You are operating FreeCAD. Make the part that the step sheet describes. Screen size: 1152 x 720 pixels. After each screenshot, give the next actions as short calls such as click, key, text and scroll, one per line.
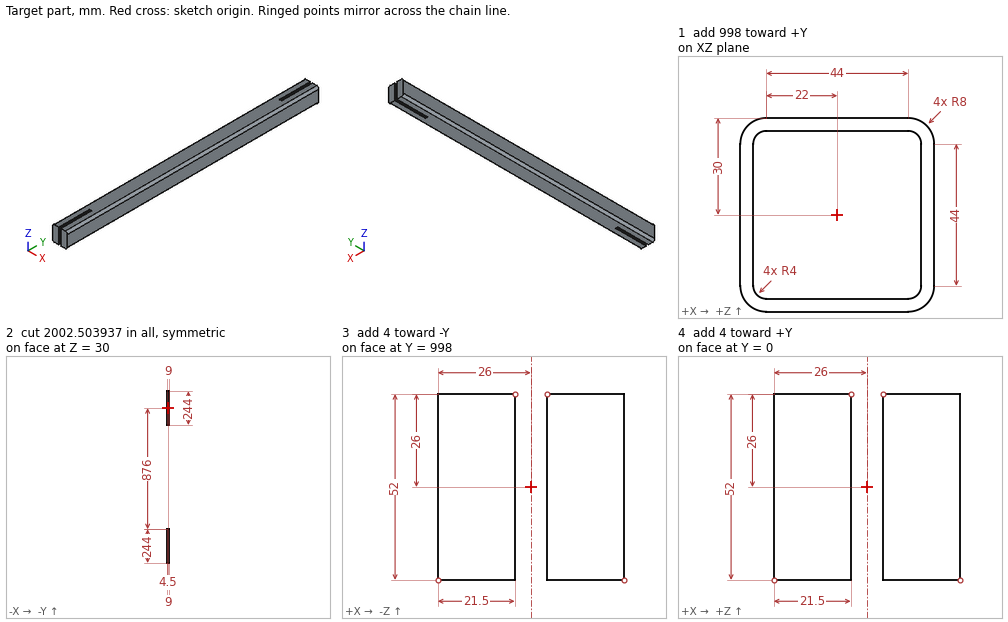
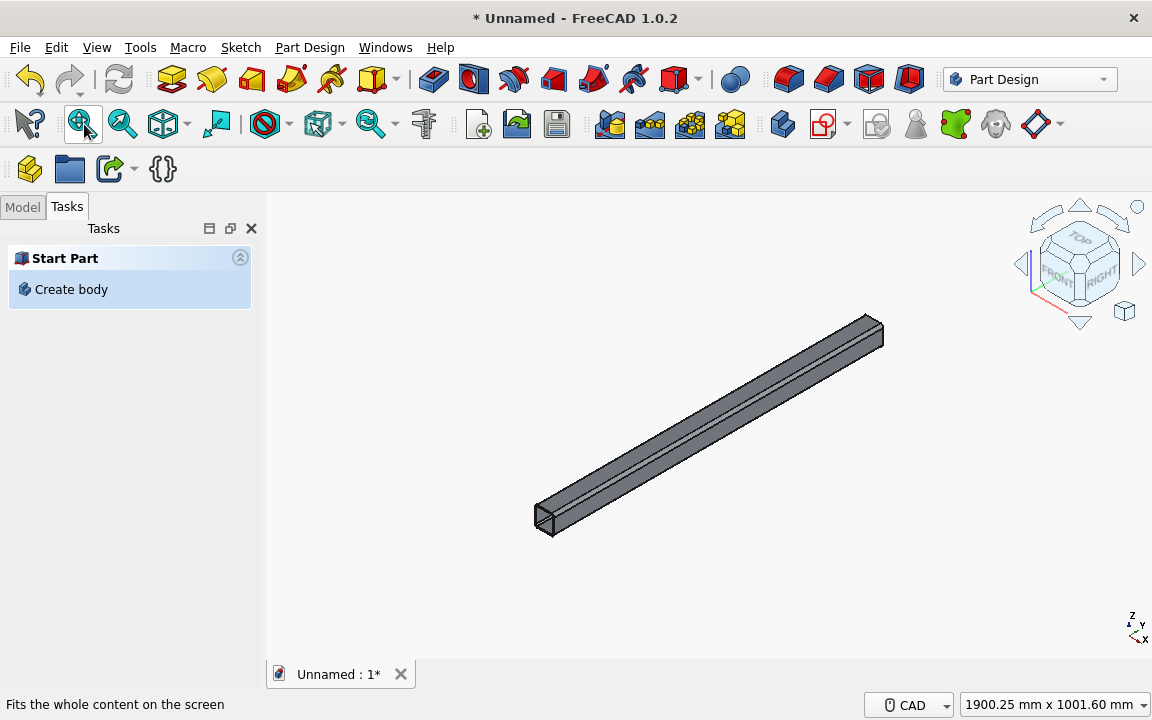
key(2)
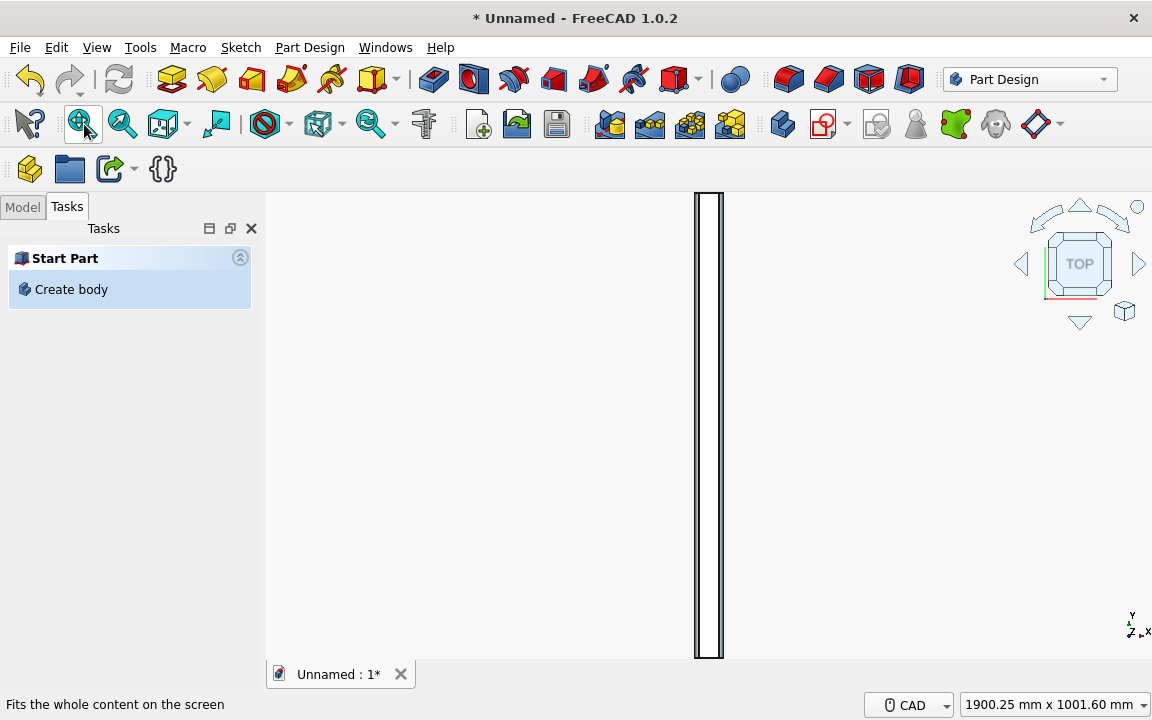
click(709, 225)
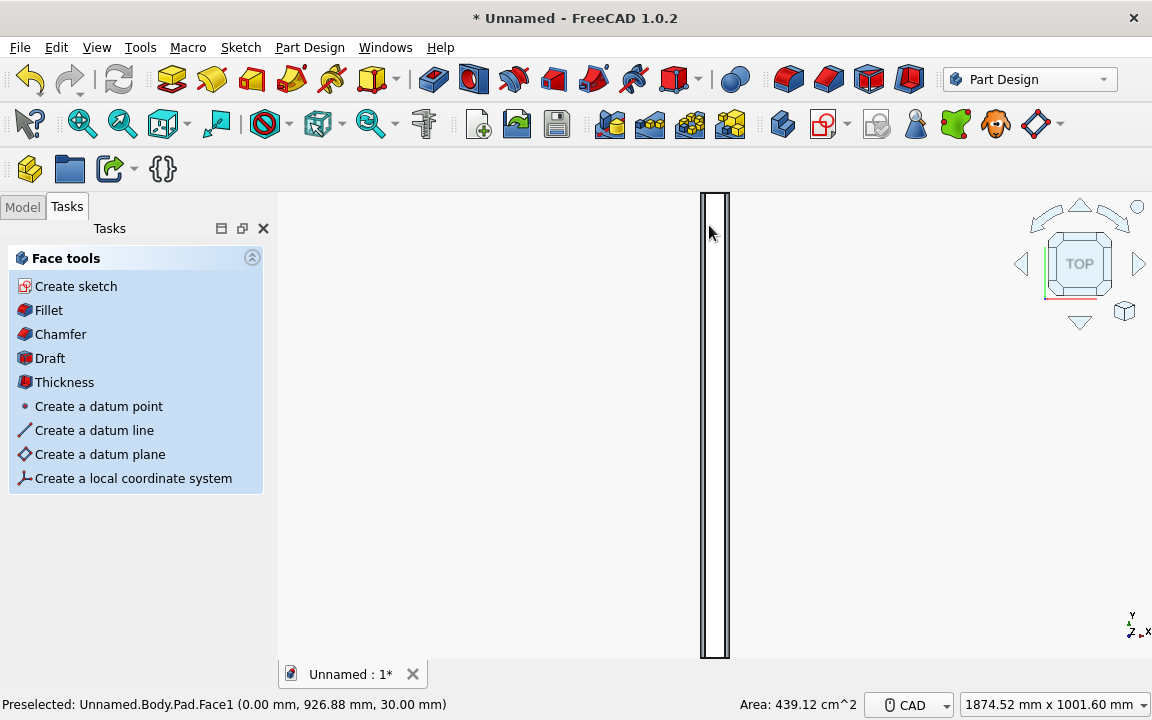
click(824, 124)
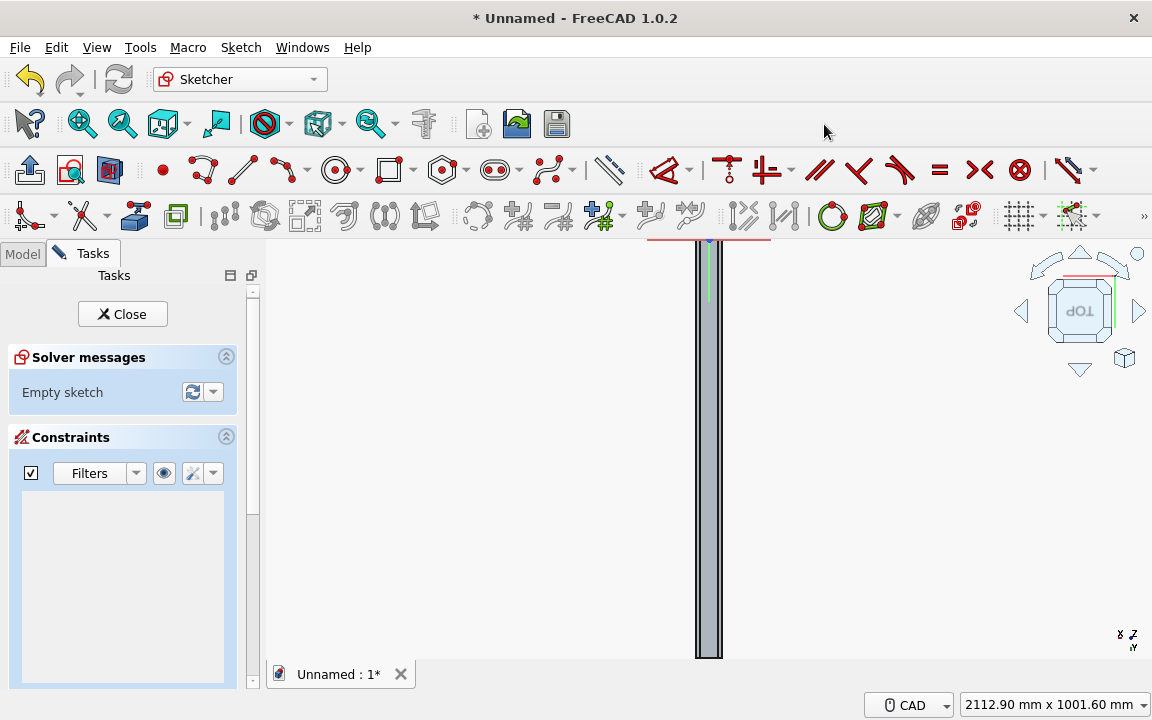
scroll(585, 449, down, 4)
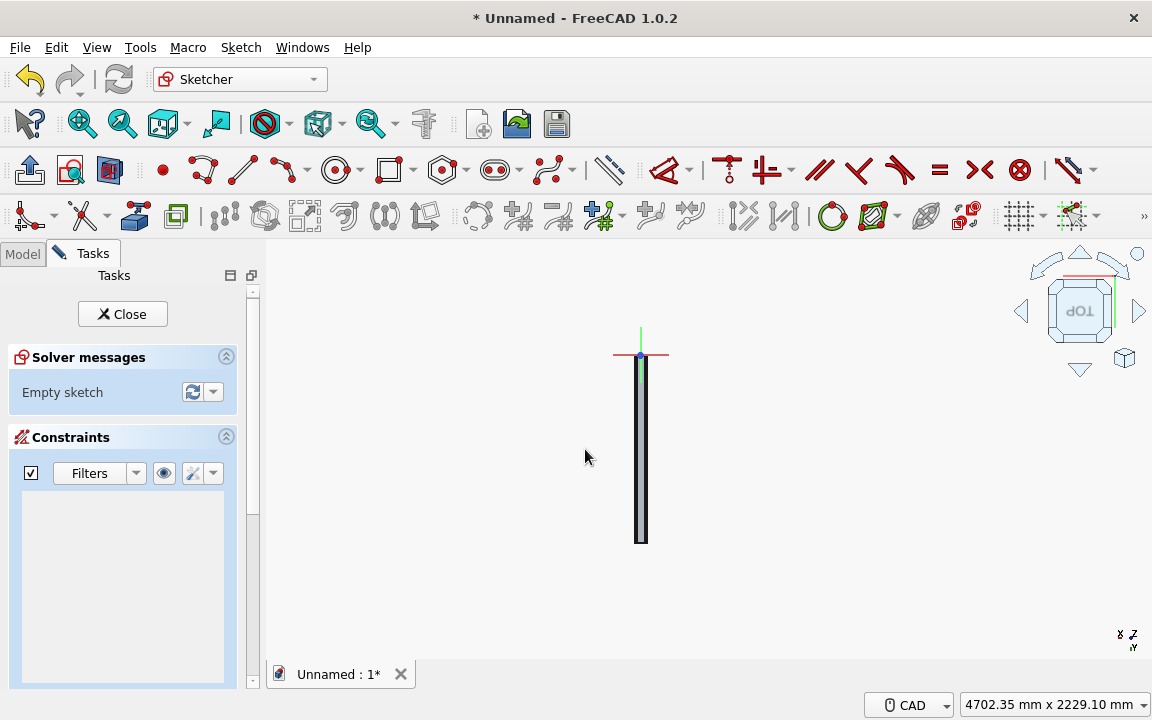
click(390, 170)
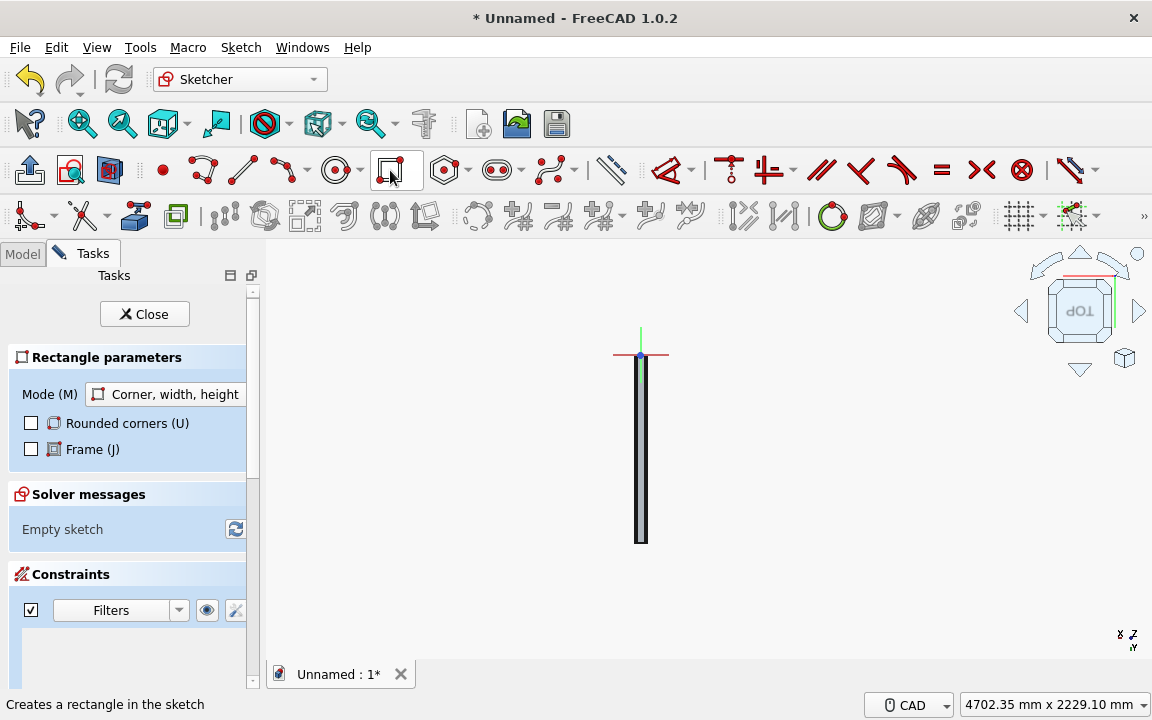
scroll(640, 520, up, 15)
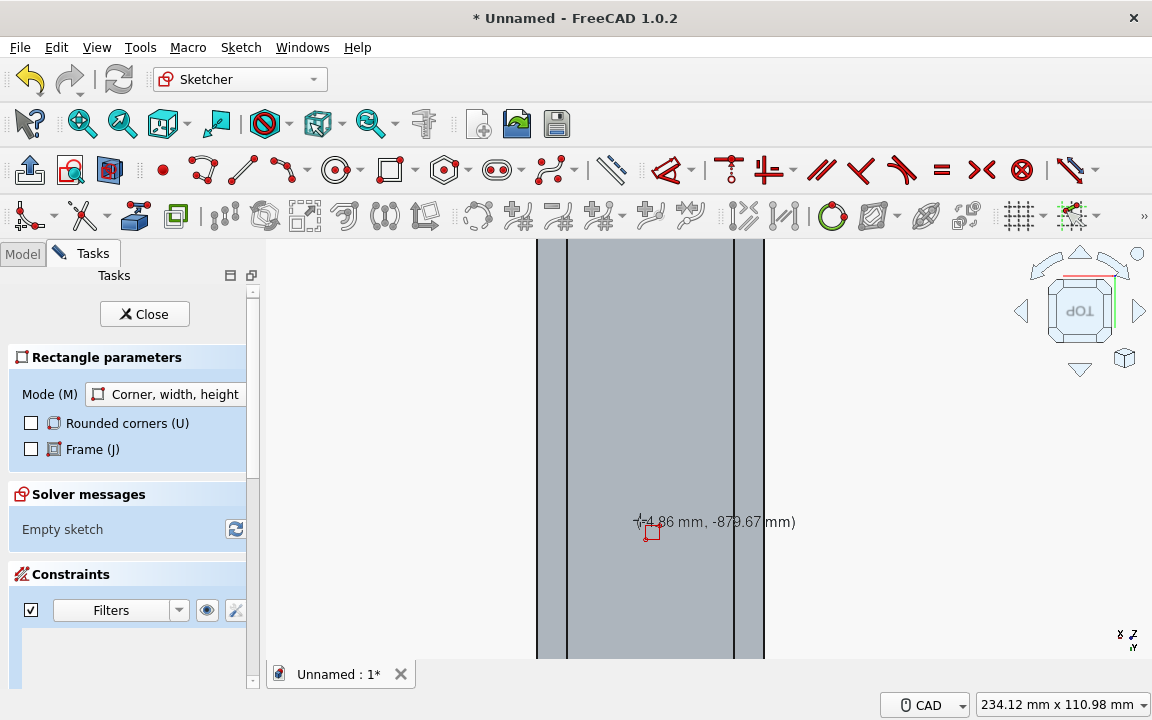
click(633, 513)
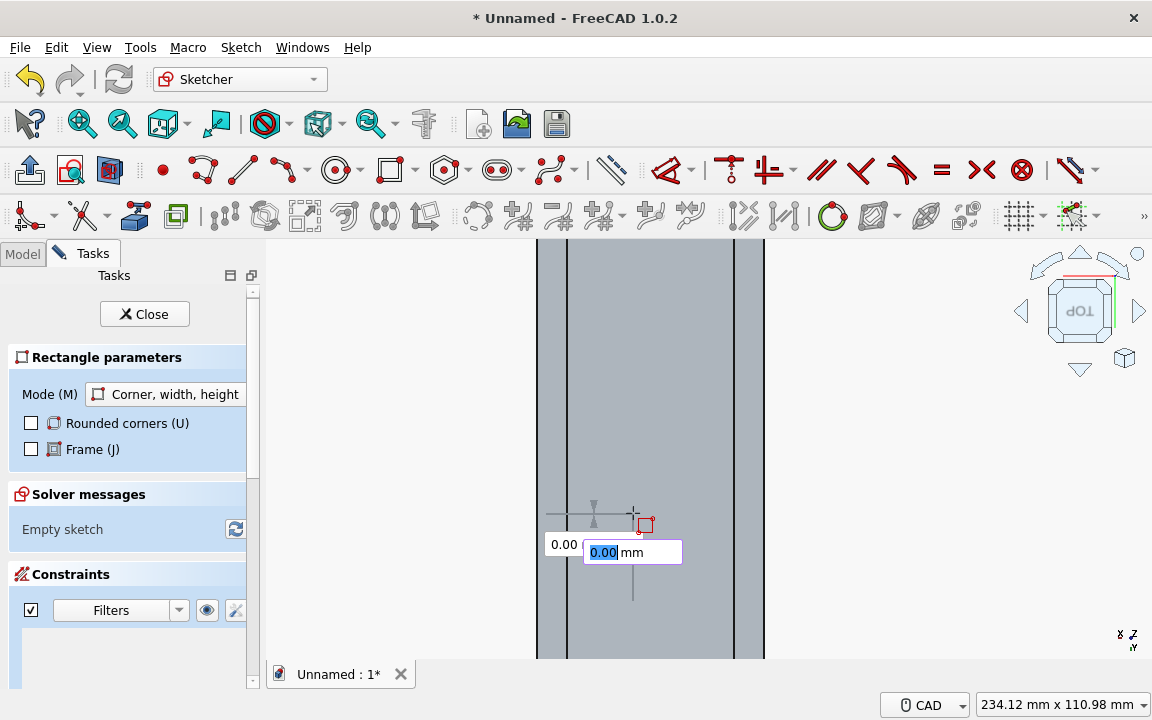
scroll(640, 520, down, 15)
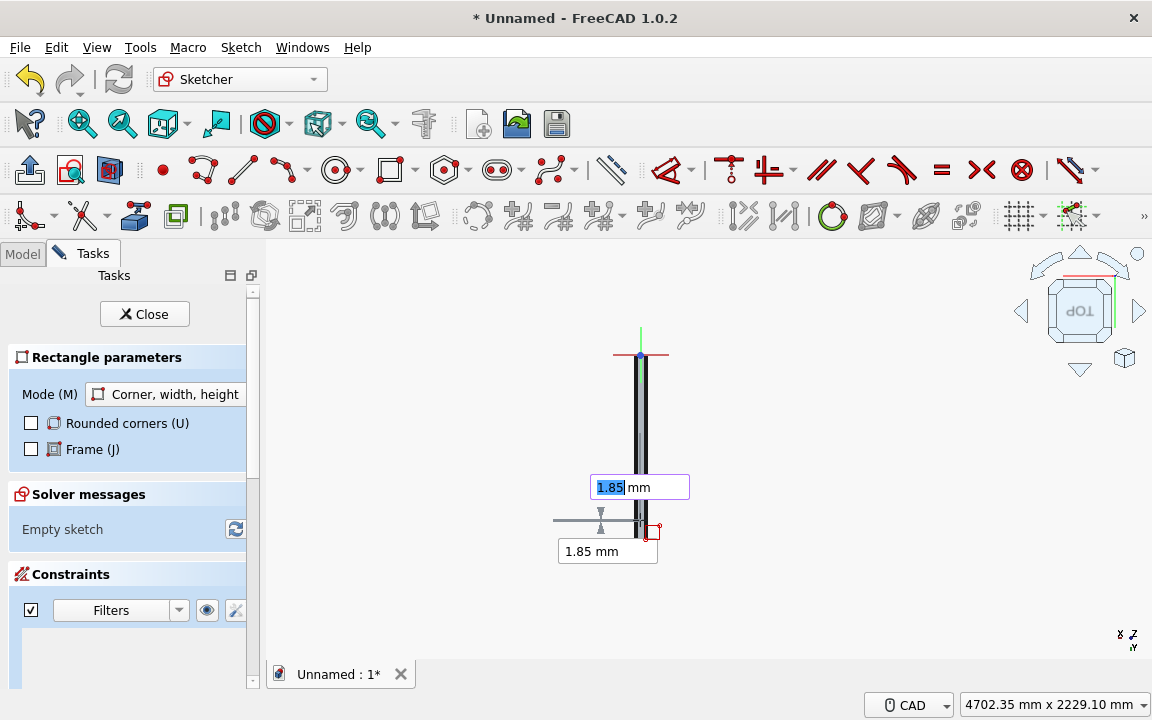
scroll(642, 566, up, 15)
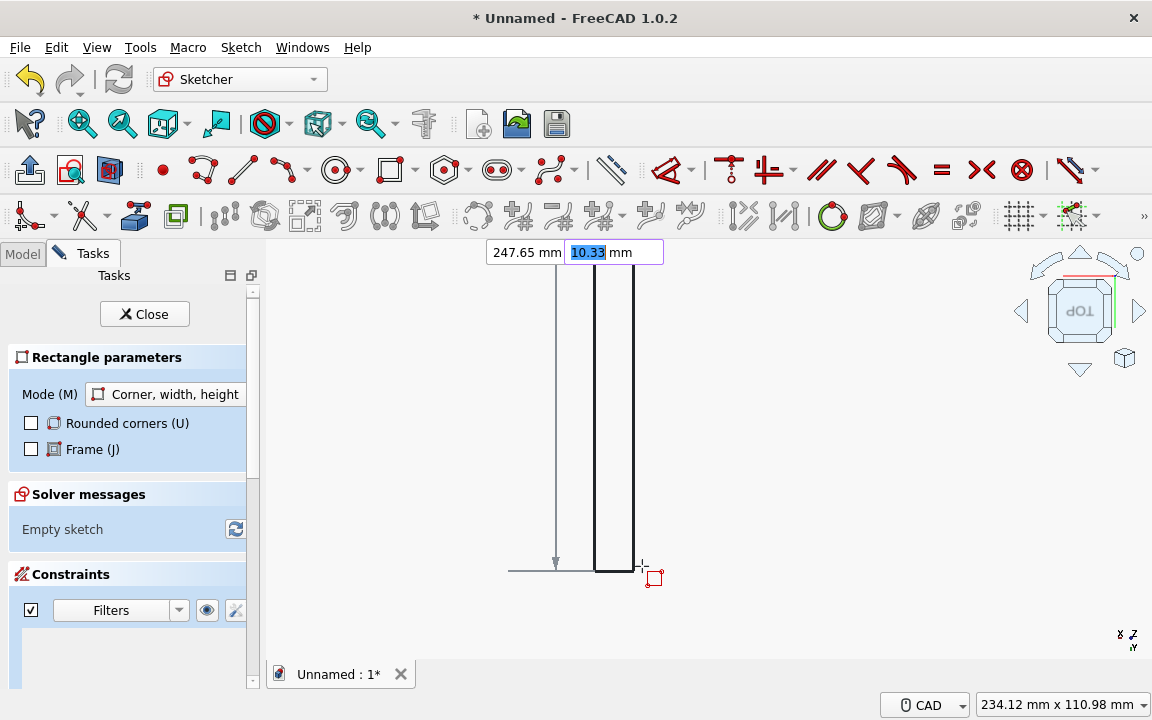
click(629, 557)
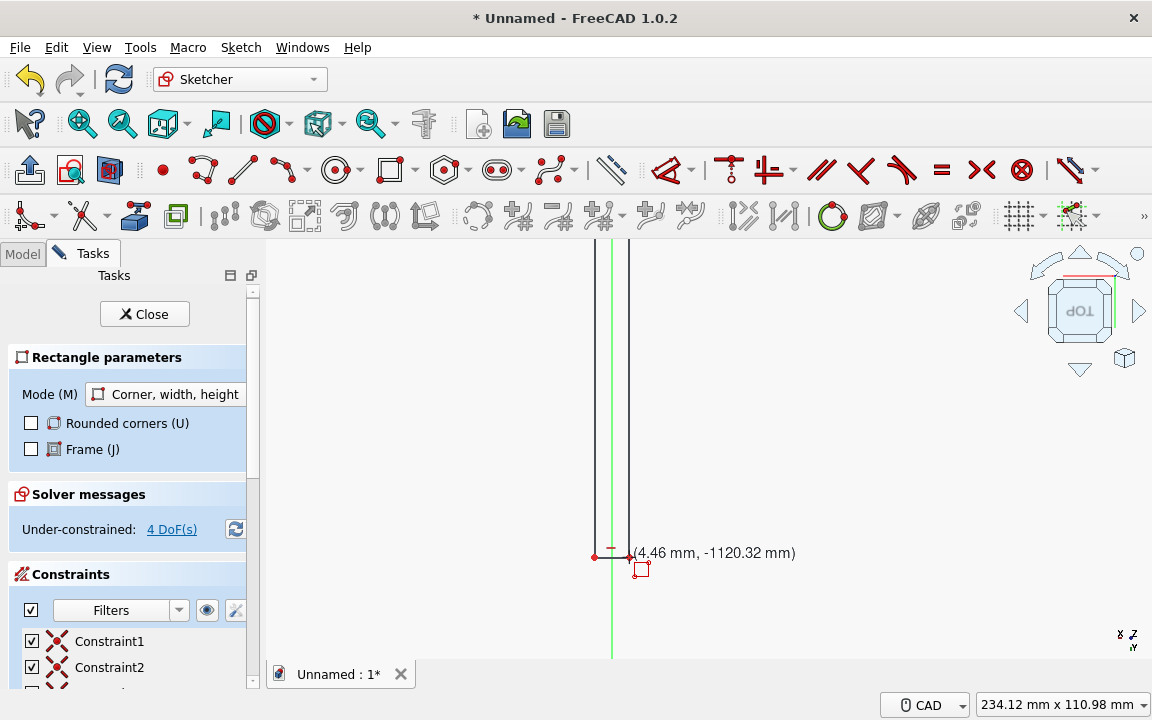
click(418, 170)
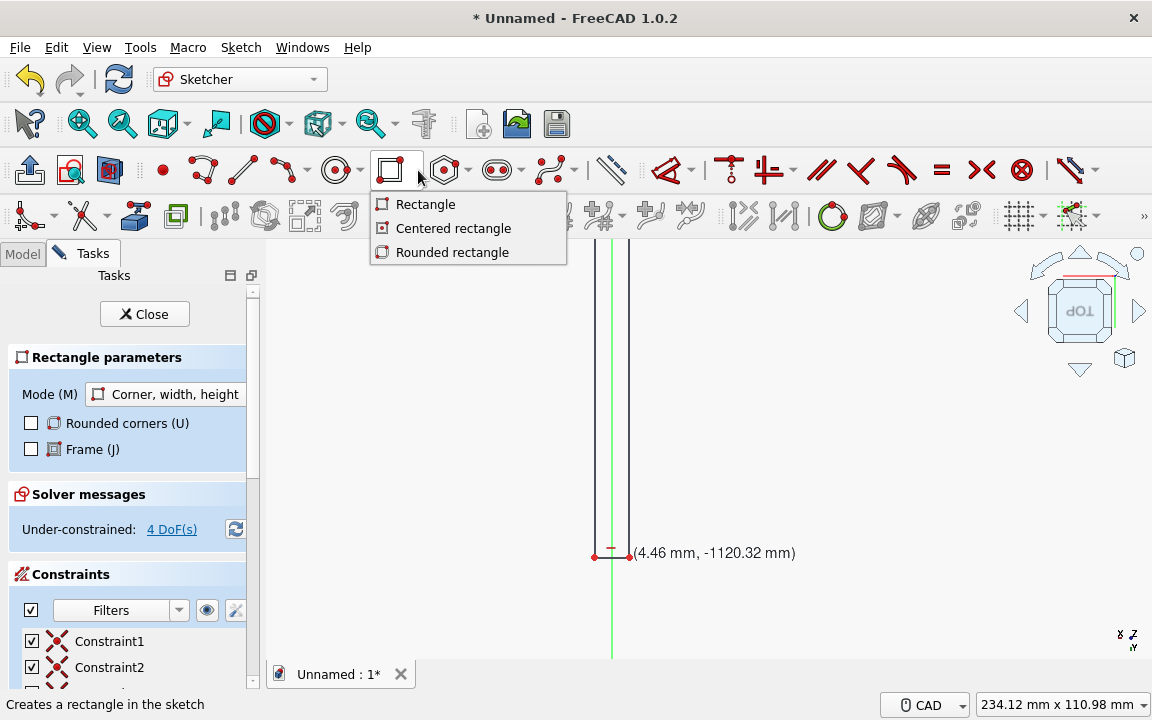
click(468, 228)